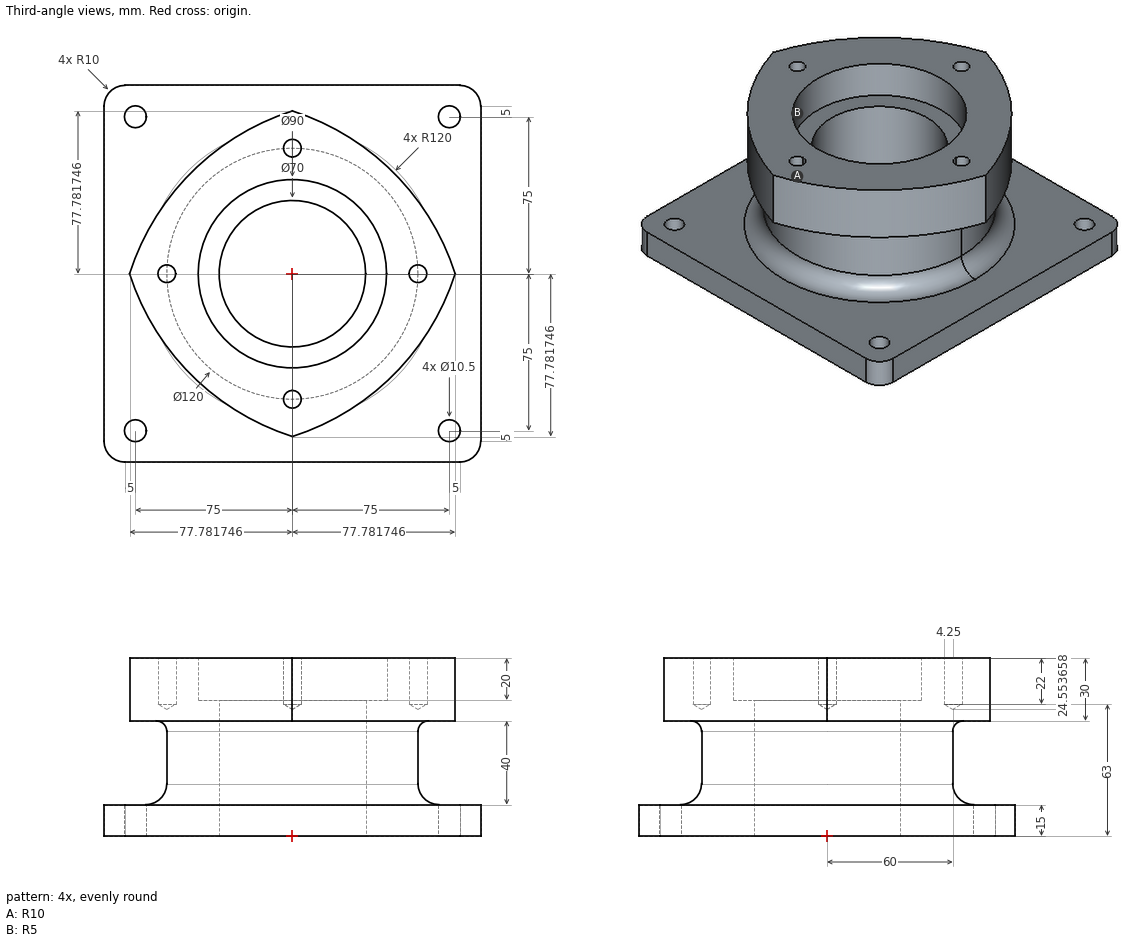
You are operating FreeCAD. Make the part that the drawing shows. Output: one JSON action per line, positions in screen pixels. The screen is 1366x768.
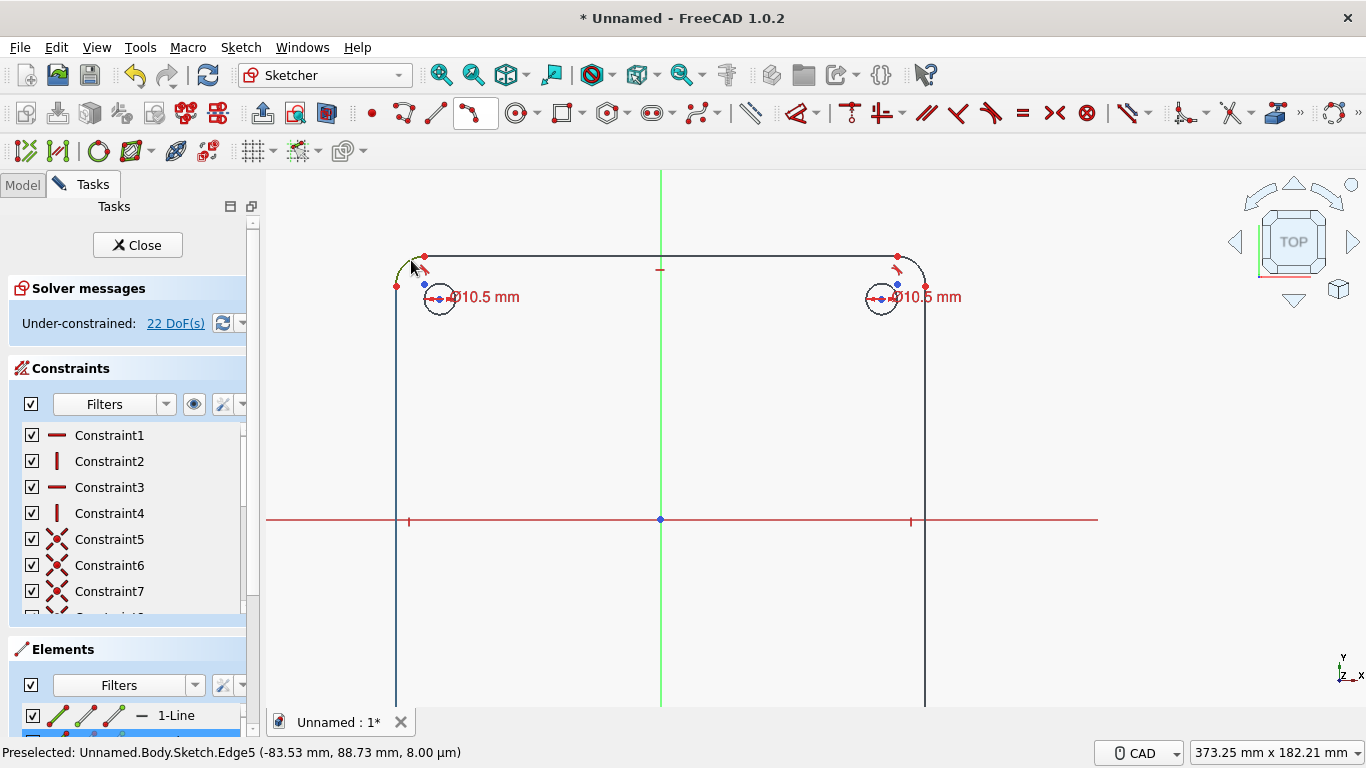
{"action": "left_click", "coordinate": [992, 114]}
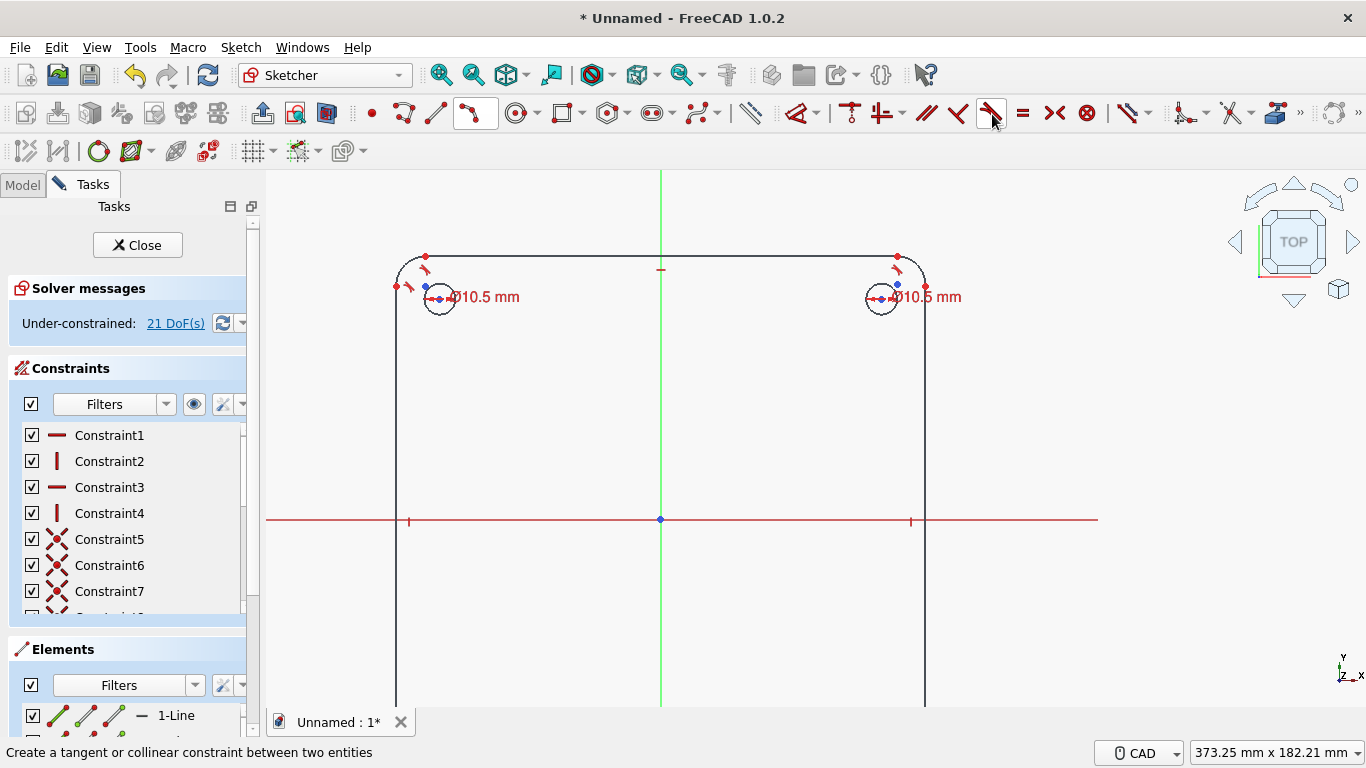
{"action": "left_click", "coordinate": [396, 427]}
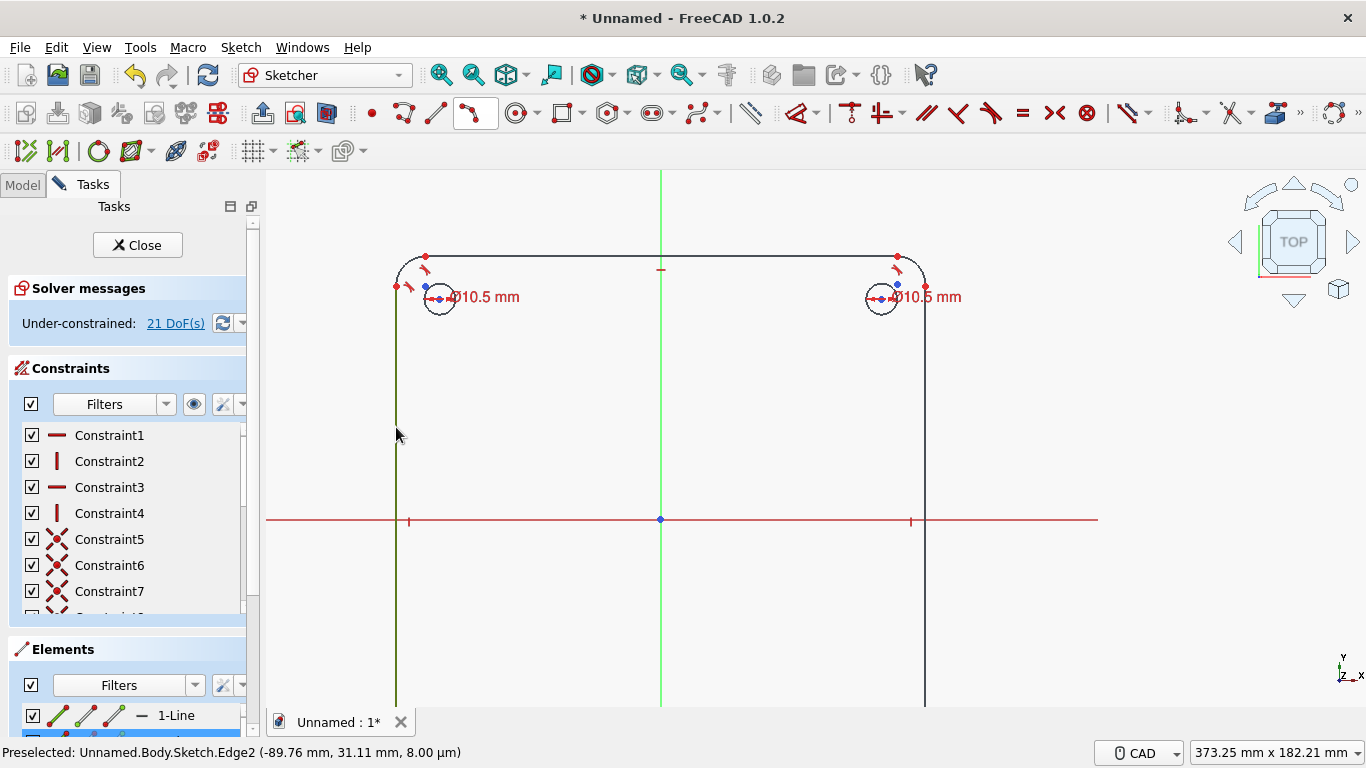
{"action": "scroll", "coordinate": [924, 273], "scroll_direction": "down", "scroll_amount": 2}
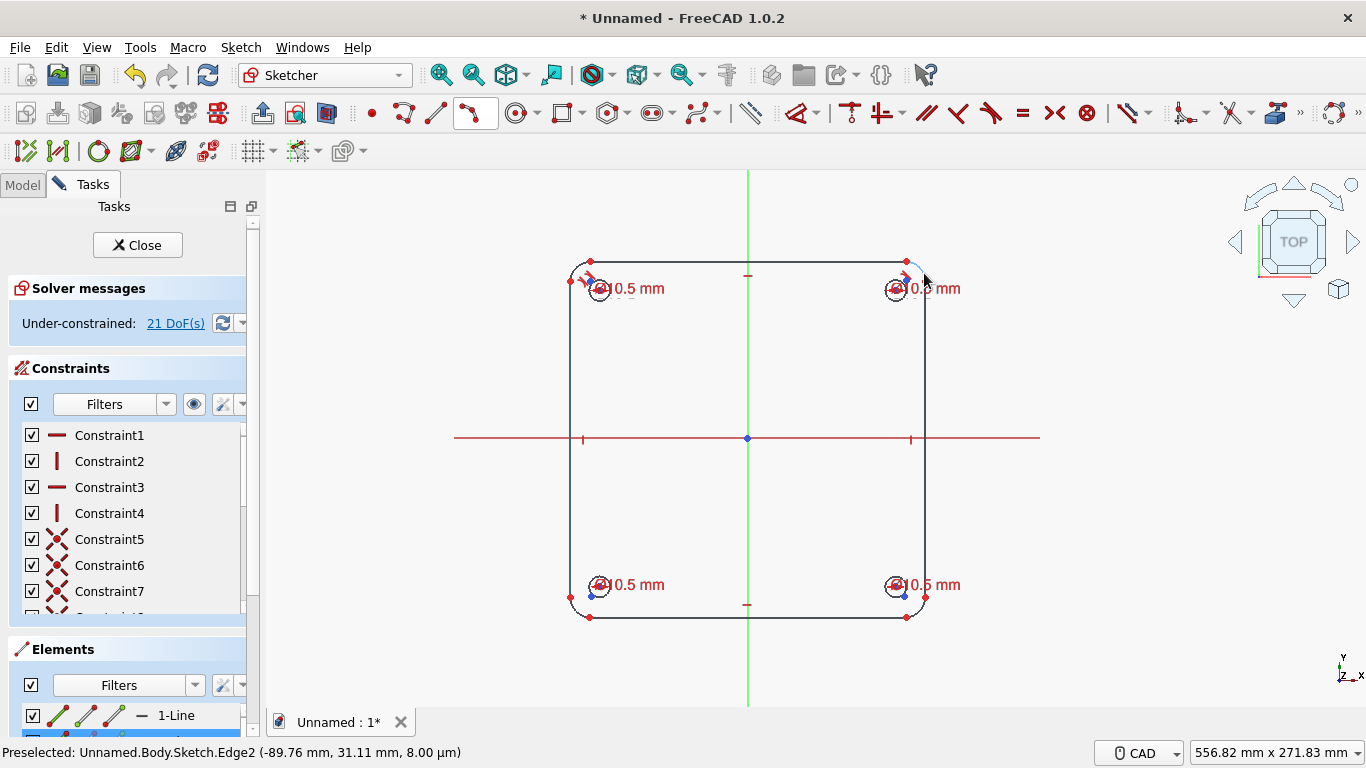
{"action": "scroll", "coordinate": [573, 606], "scroll_direction": "up", "scroll_amount": 3}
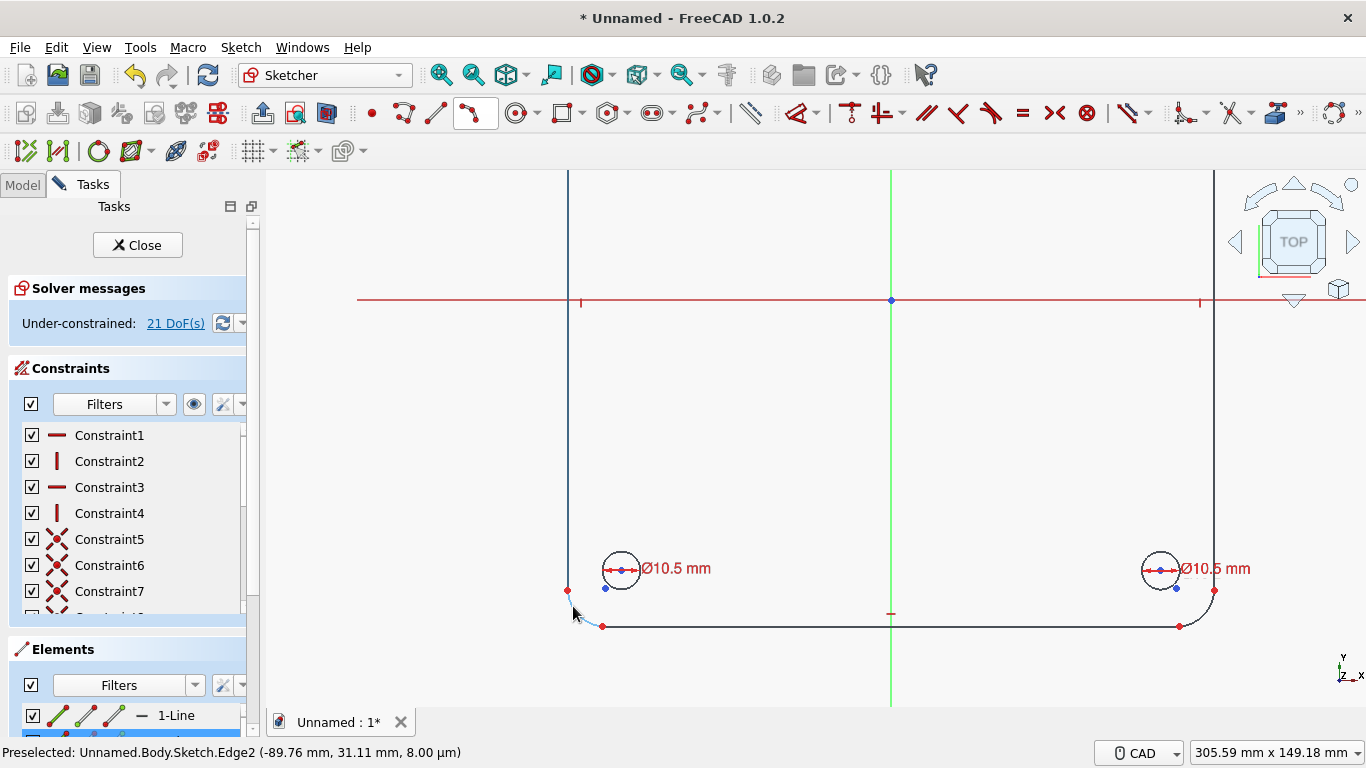
{"action": "left_click", "coordinate": [572, 606]}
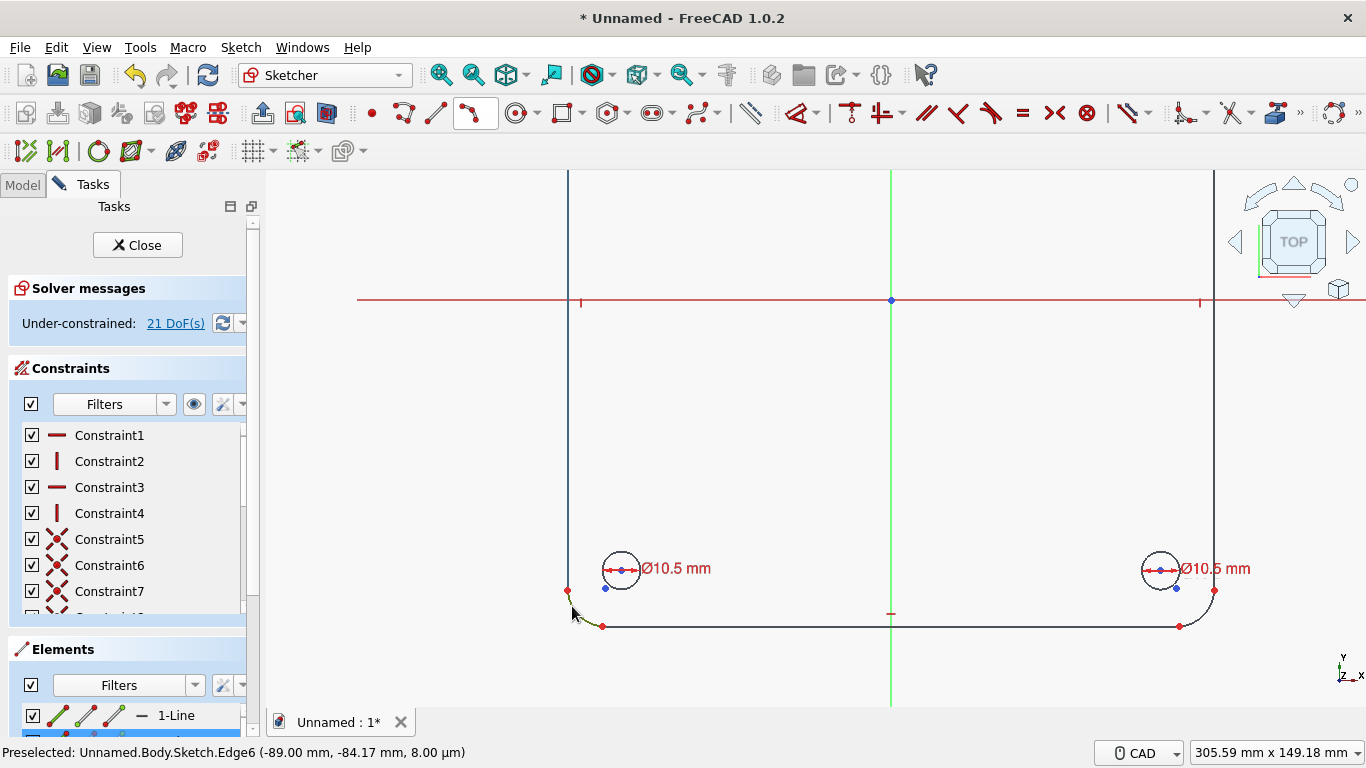
{"action": "left_click", "coordinate": [992, 114]}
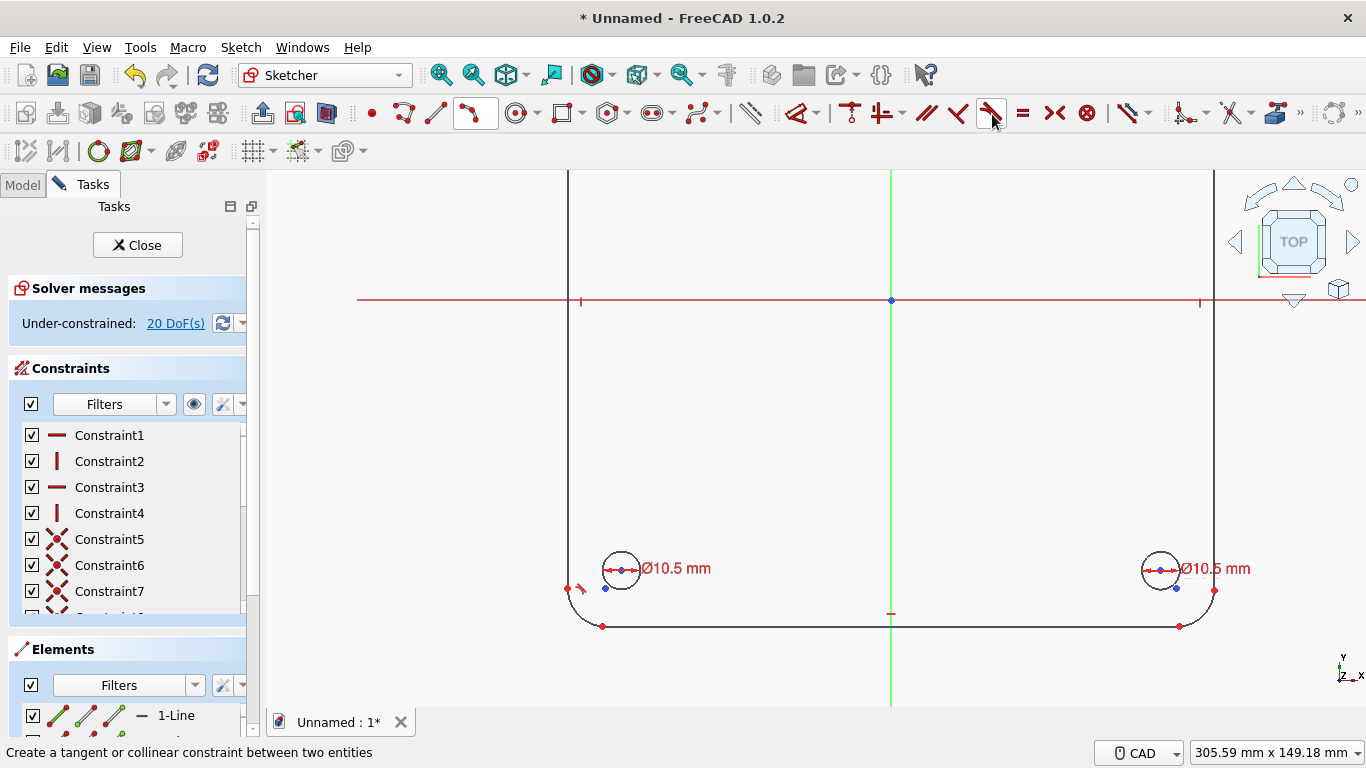
{"action": "left_click", "coordinate": [776, 627]}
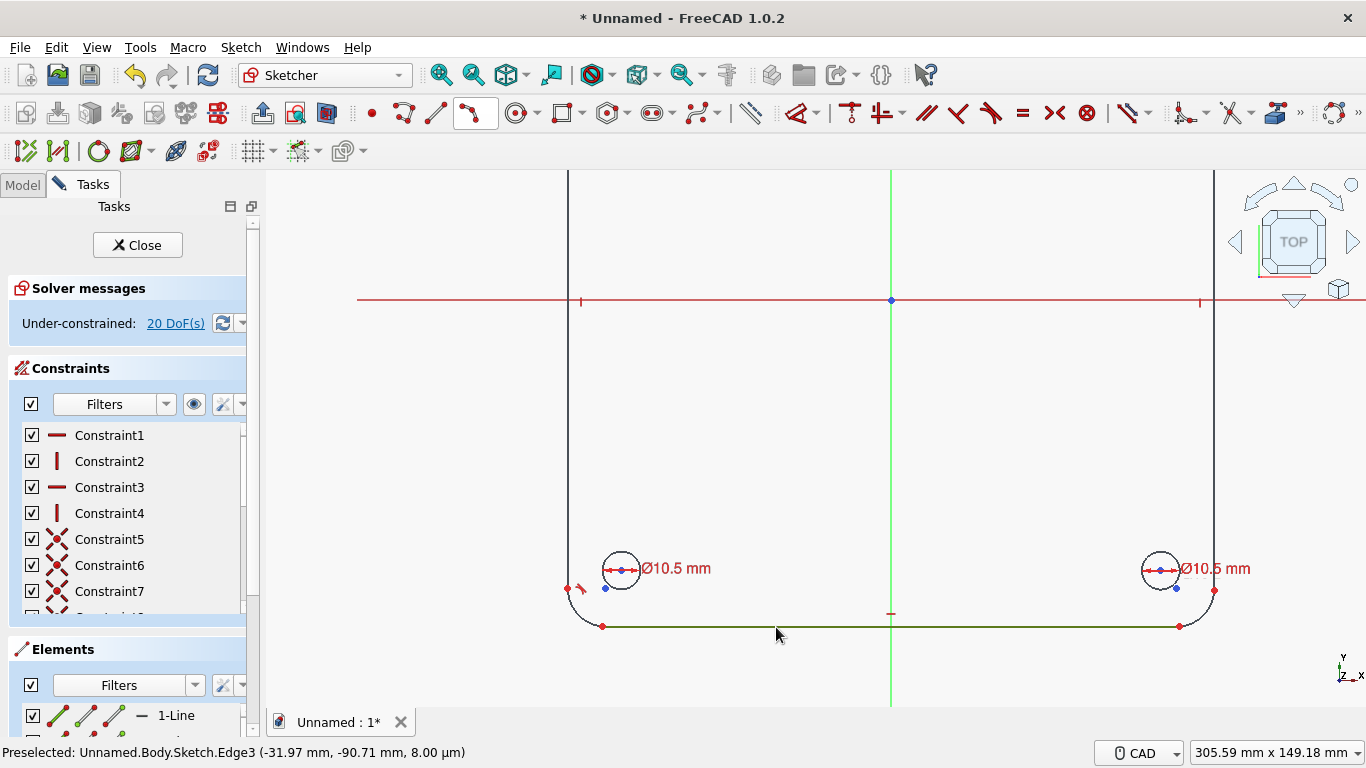
{"action": "left_click", "coordinate": [572, 605]}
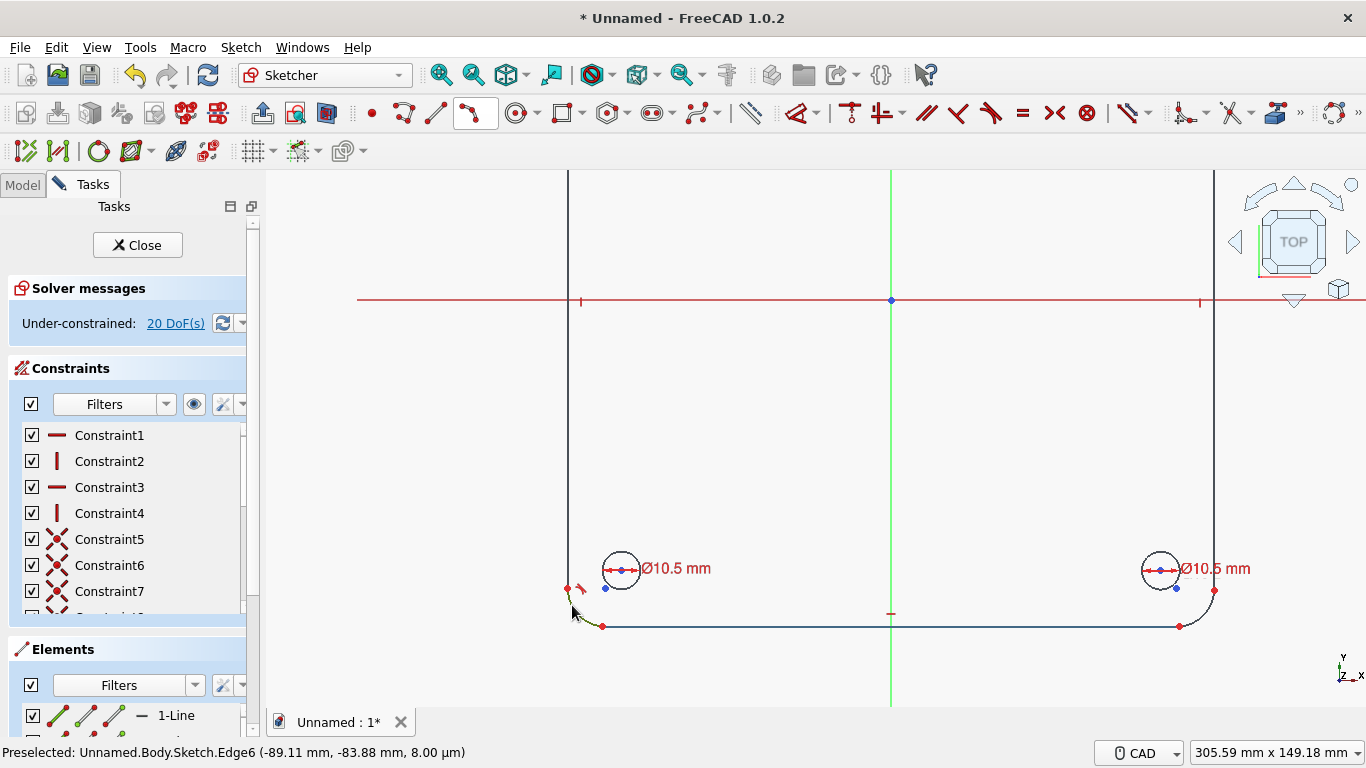
{"action": "left_click", "coordinate": [992, 114]}